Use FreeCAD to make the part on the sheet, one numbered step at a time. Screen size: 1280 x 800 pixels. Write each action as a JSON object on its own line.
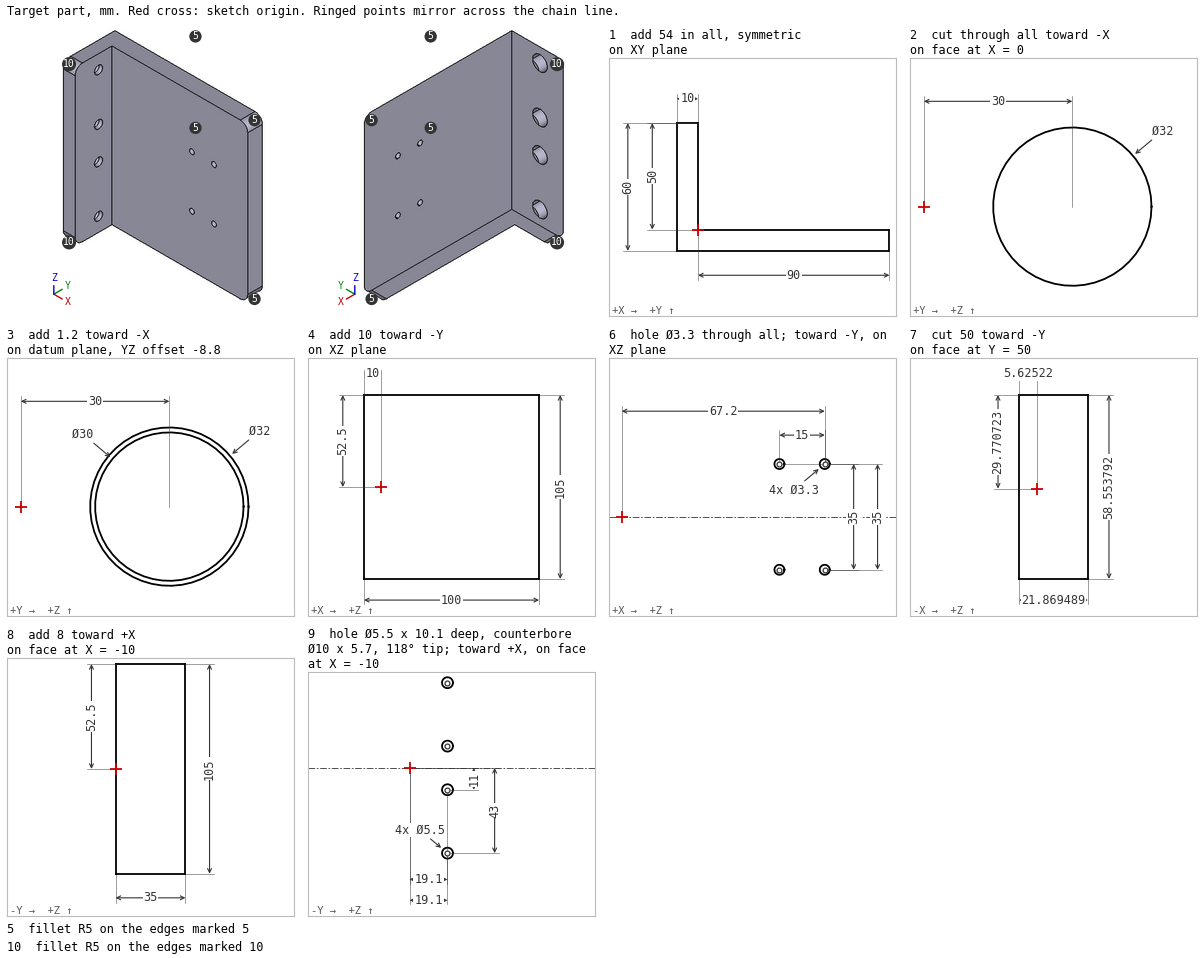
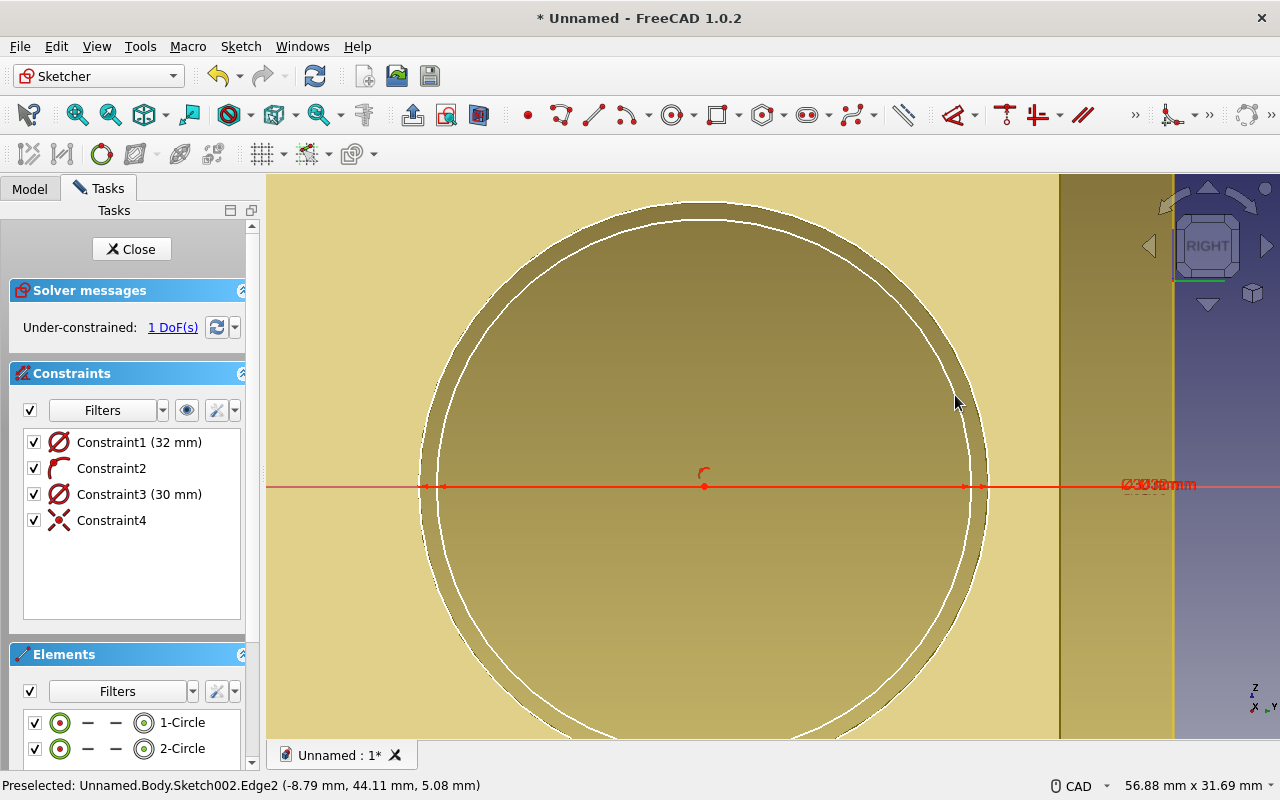
{"action": "left_click", "coordinate": [952, 116]}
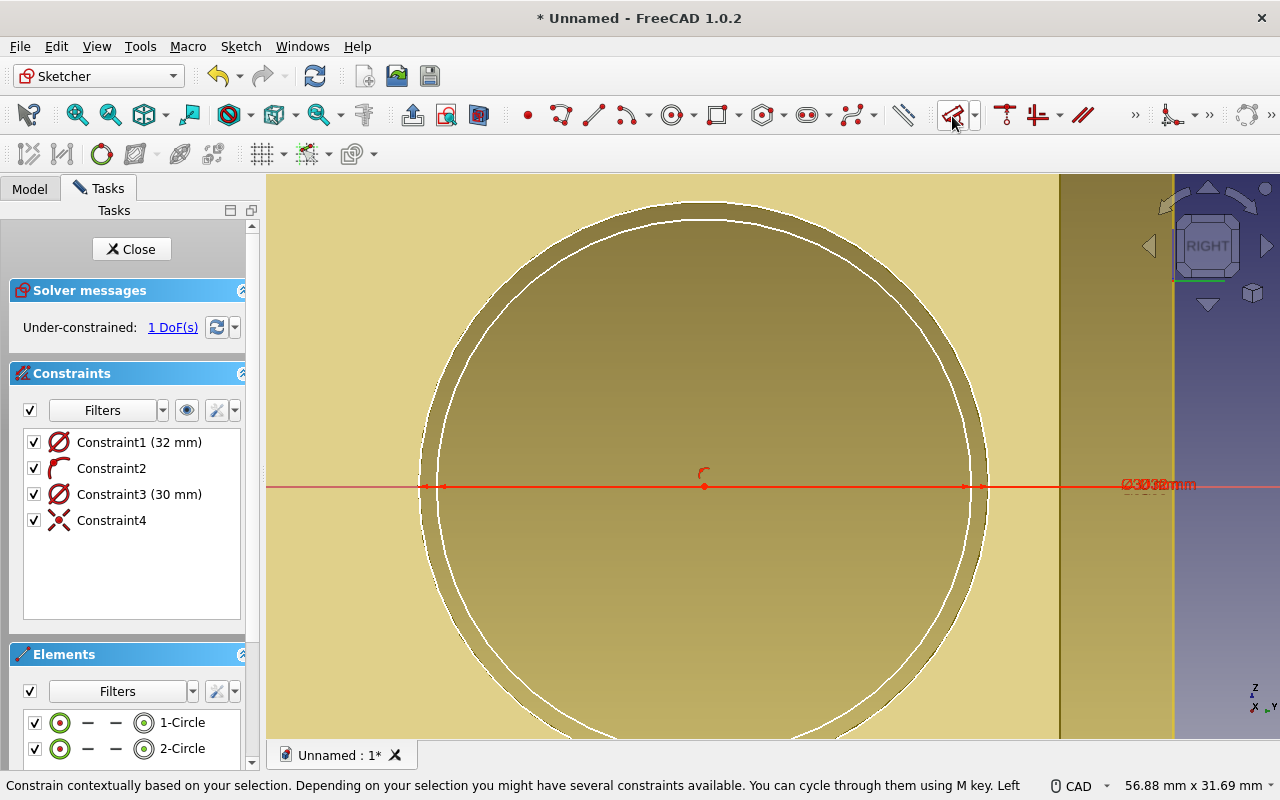
{"action": "left_click", "coordinate": [704, 487]}
{"action": "left_click", "coordinate": [499, 521]}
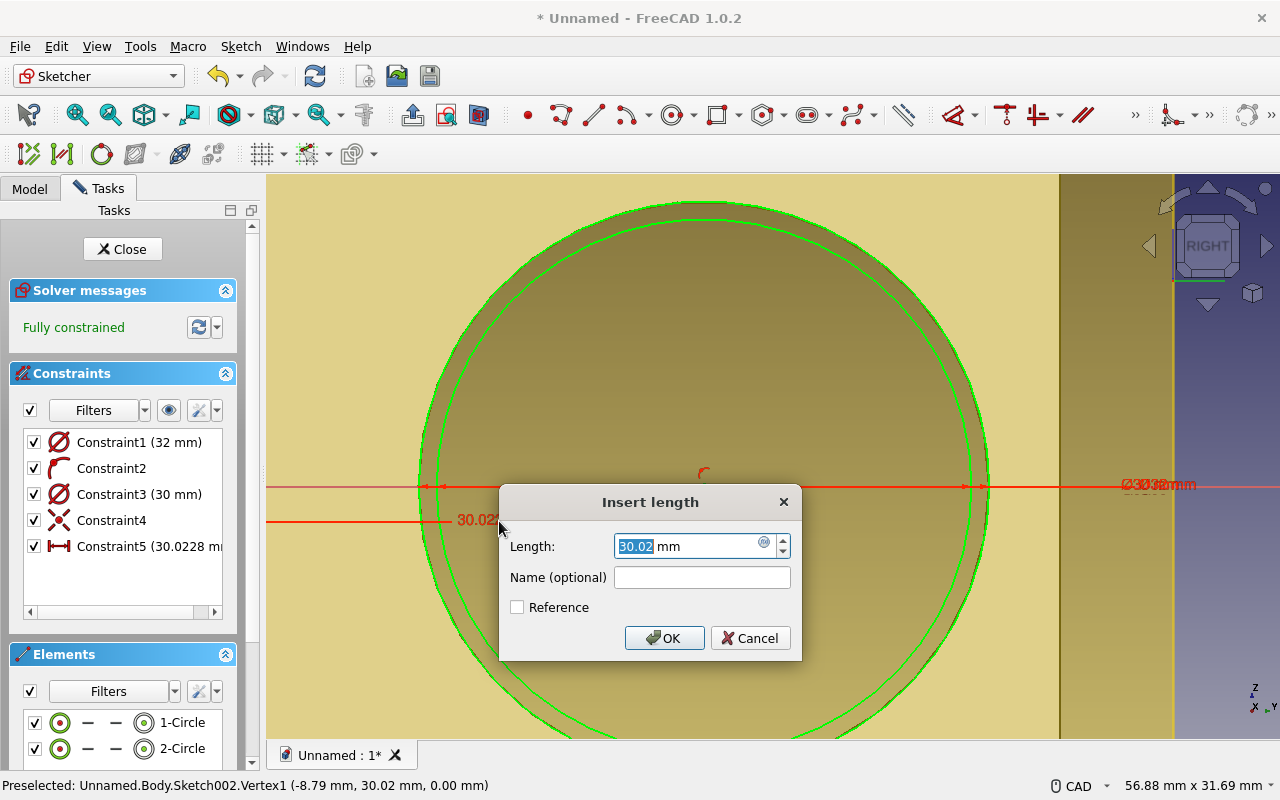
{"action": "type", "text": "30"}
{"action": "key", "text": "Return"}
{"action": "key", "text": "Escape"}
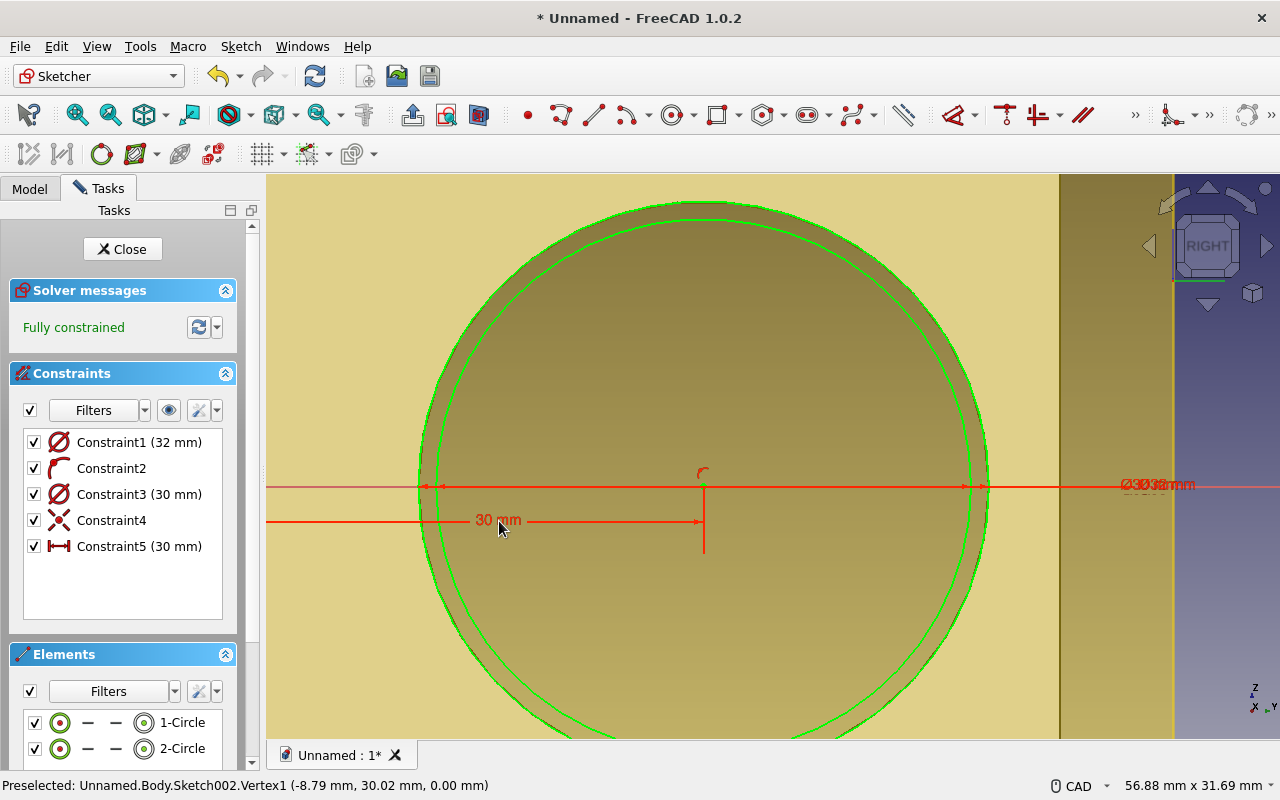
{"action": "left_click", "coordinate": [123, 249]}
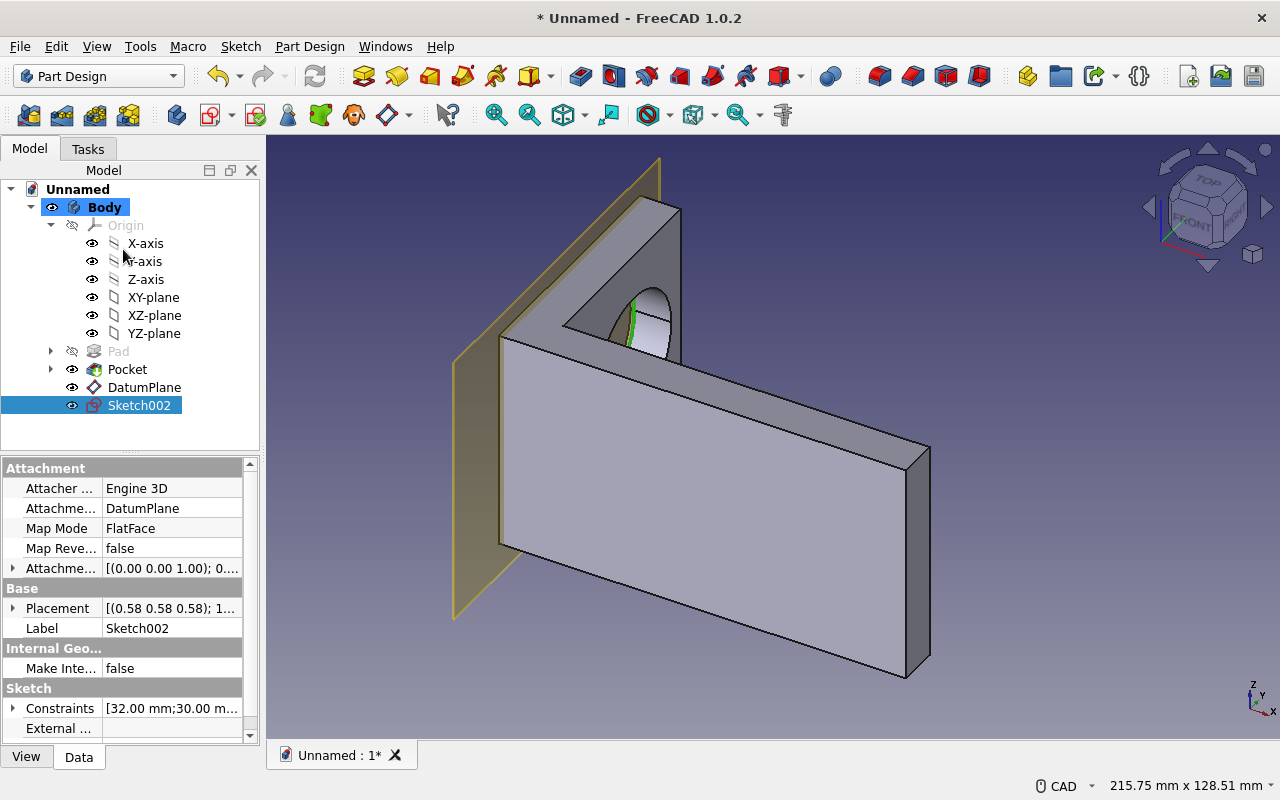
{"action": "left_click", "coordinate": [364, 76]}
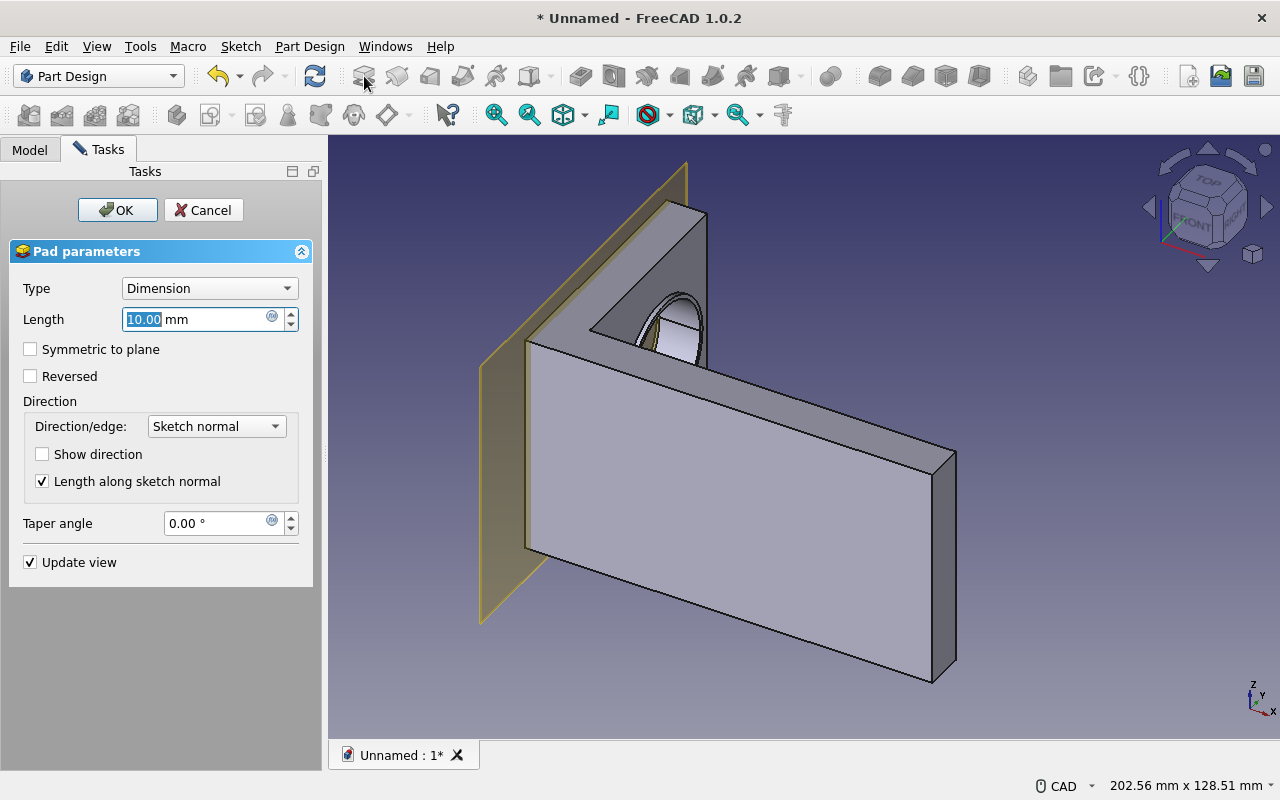
{"action": "type", "text": "1.2"}
{"action": "key", "text": "Tab"}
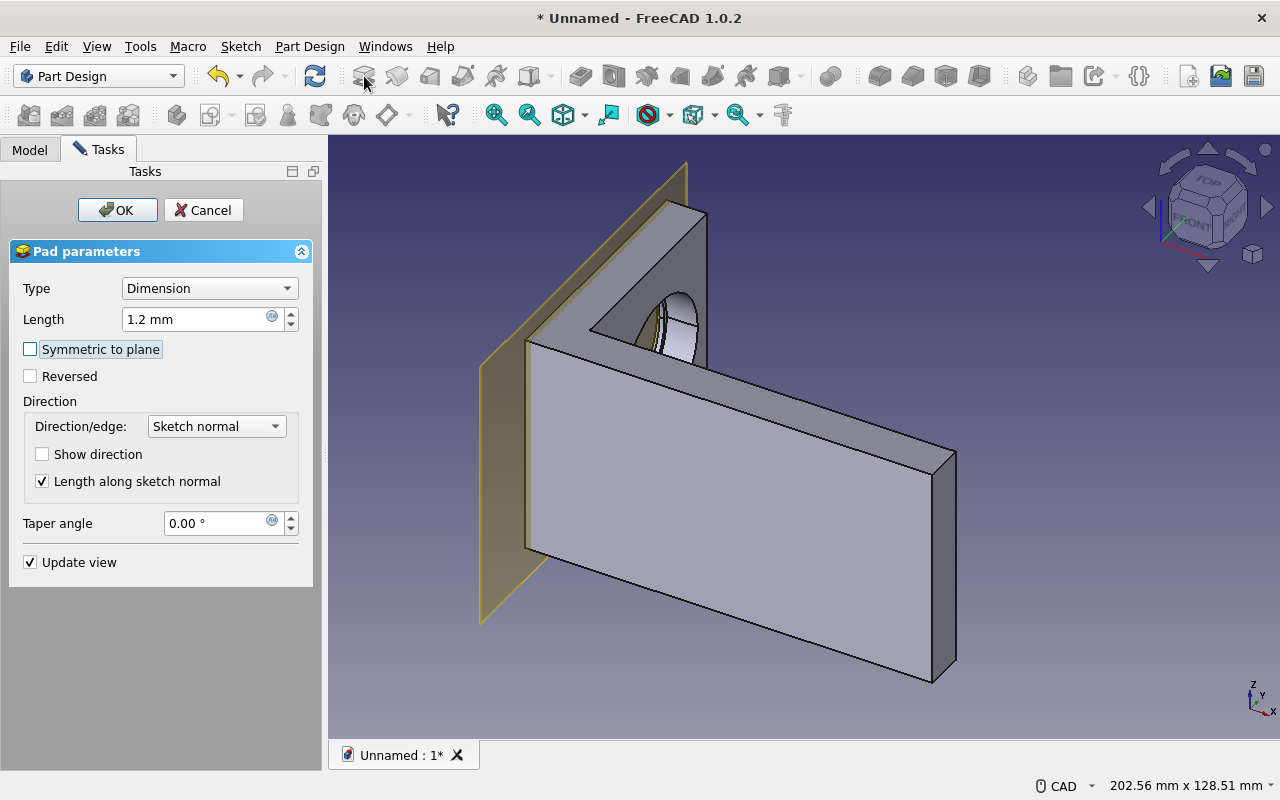
{"action": "left_click", "coordinate": [31, 376]}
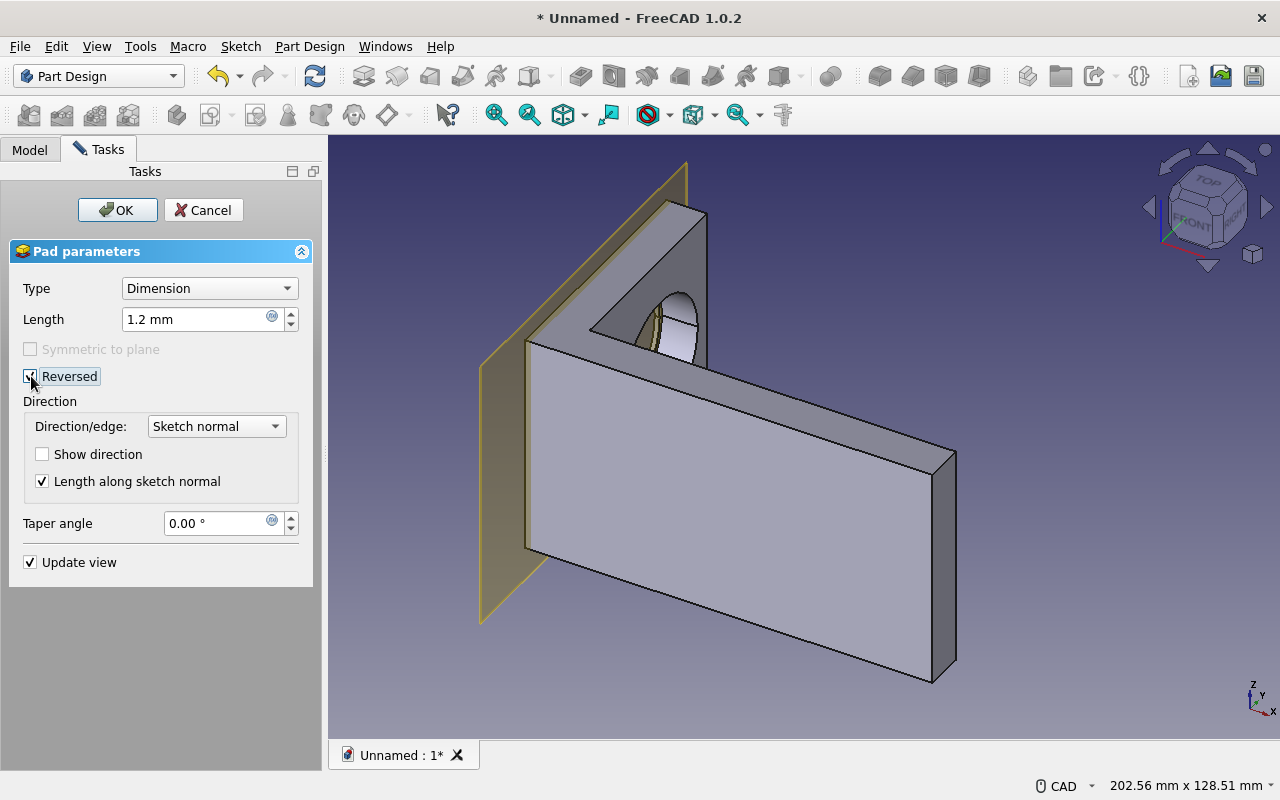
{"action": "left_click", "coordinate": [118, 210]}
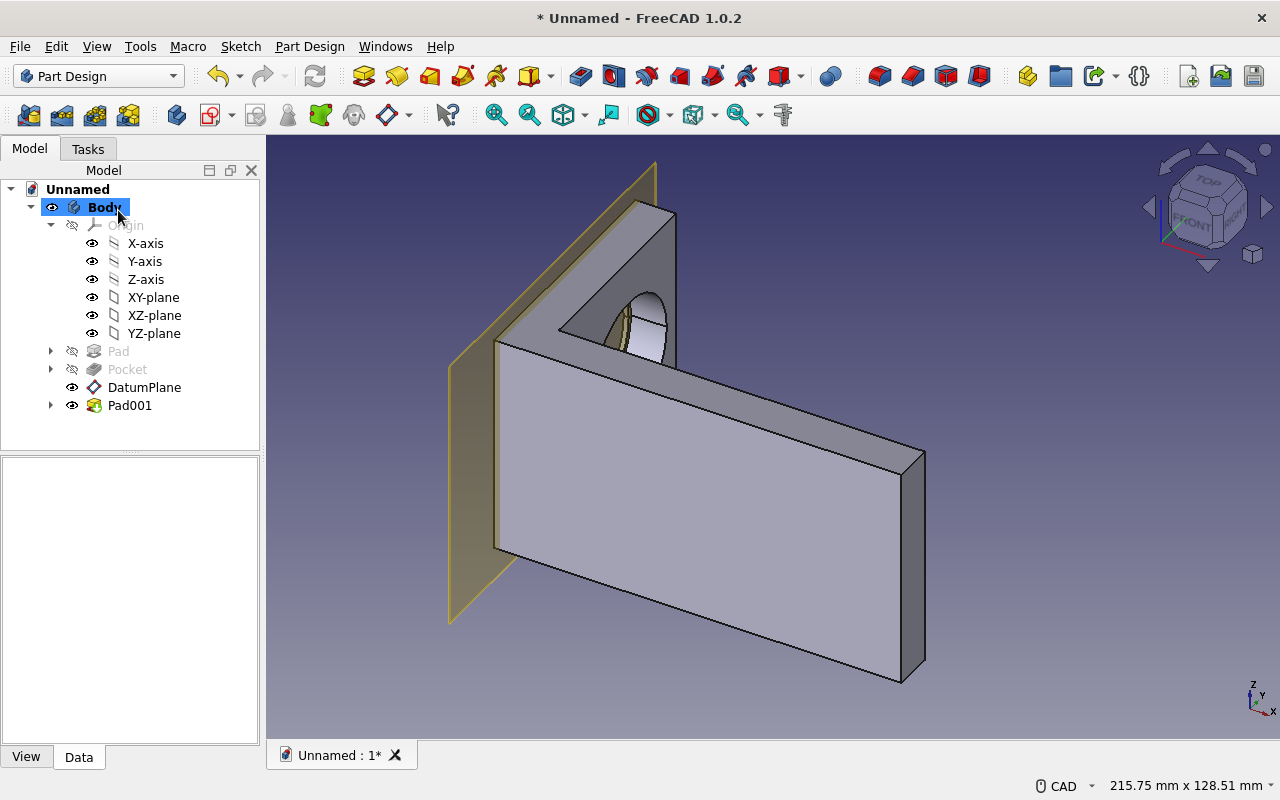
{"action": "left_click", "coordinate": [117, 387]}
{"action": "key", "text": "space"}